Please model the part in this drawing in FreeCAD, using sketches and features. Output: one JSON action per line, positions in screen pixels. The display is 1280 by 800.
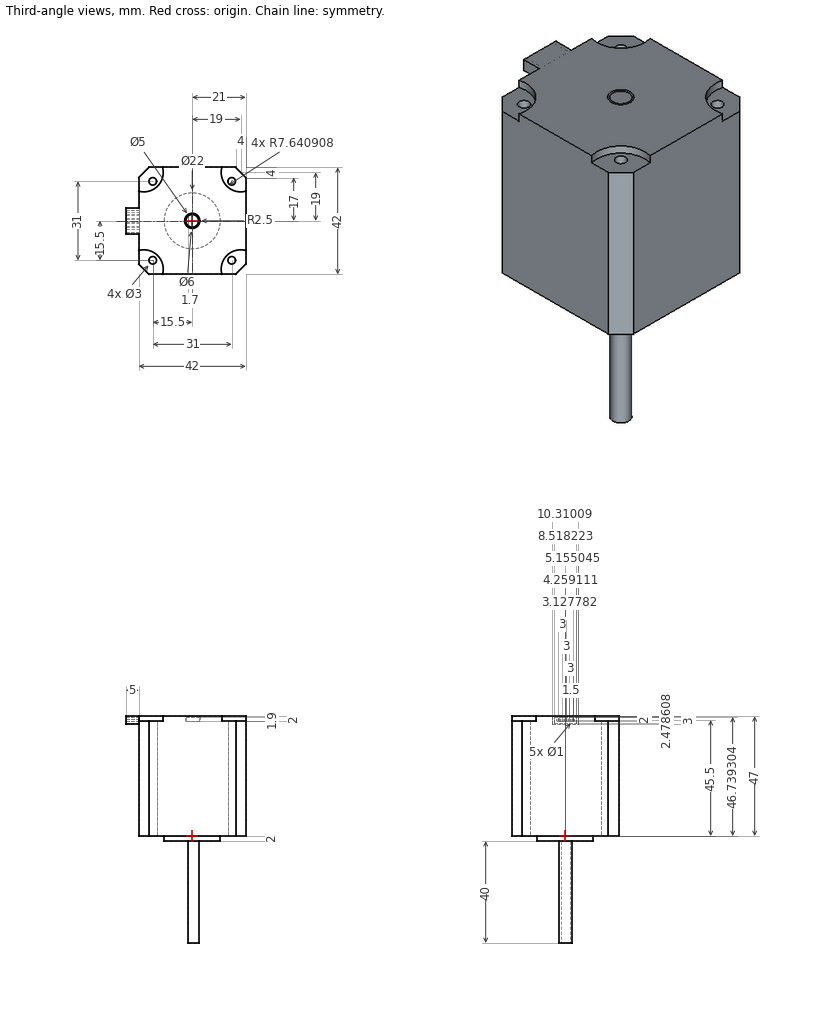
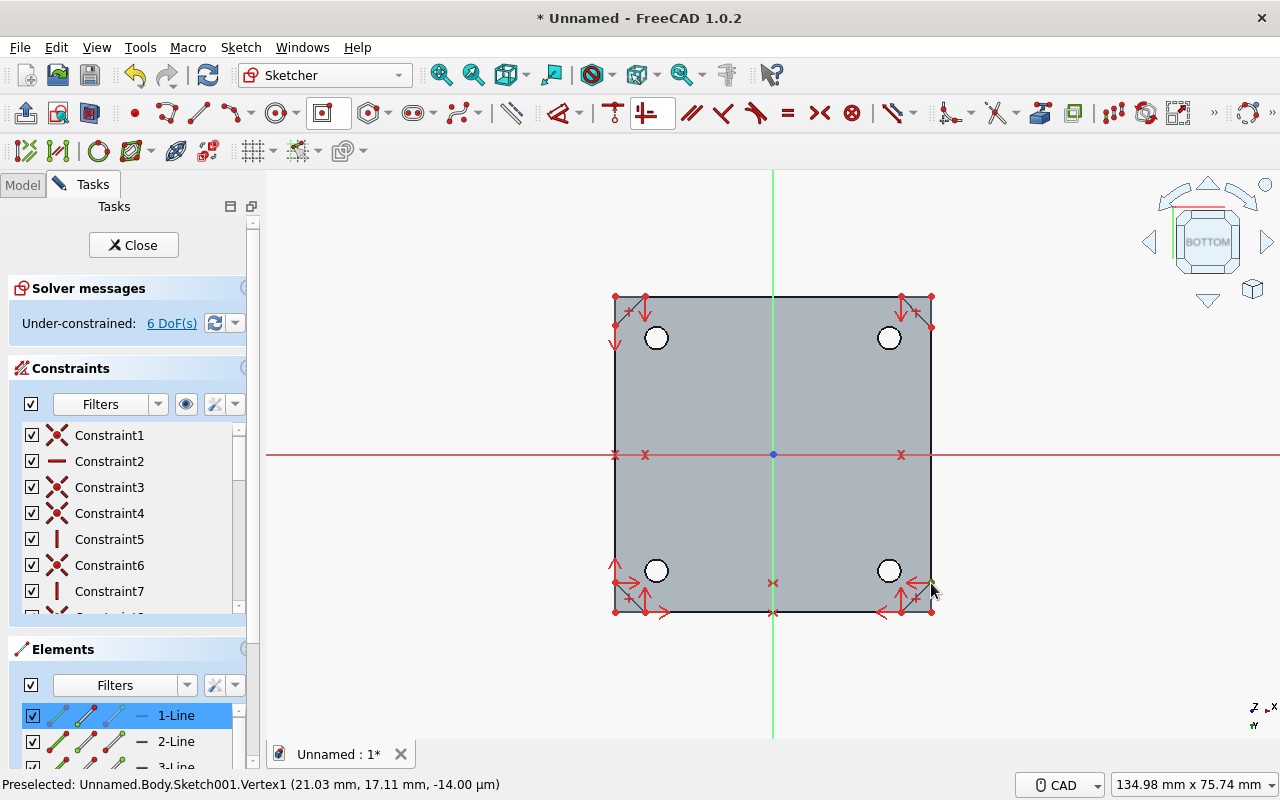
{"action": "left_click", "coordinate": [931, 328]}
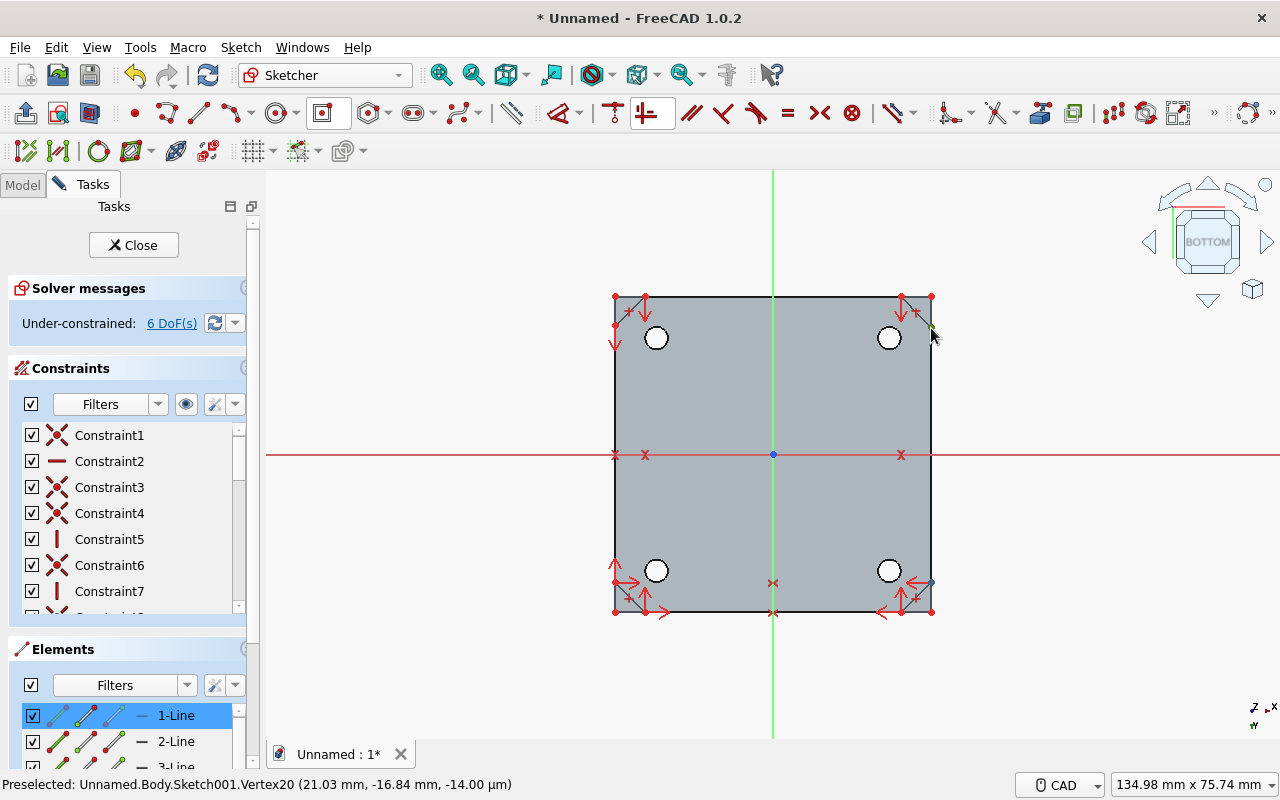
{"action": "left_click", "coordinate": [353, 454]}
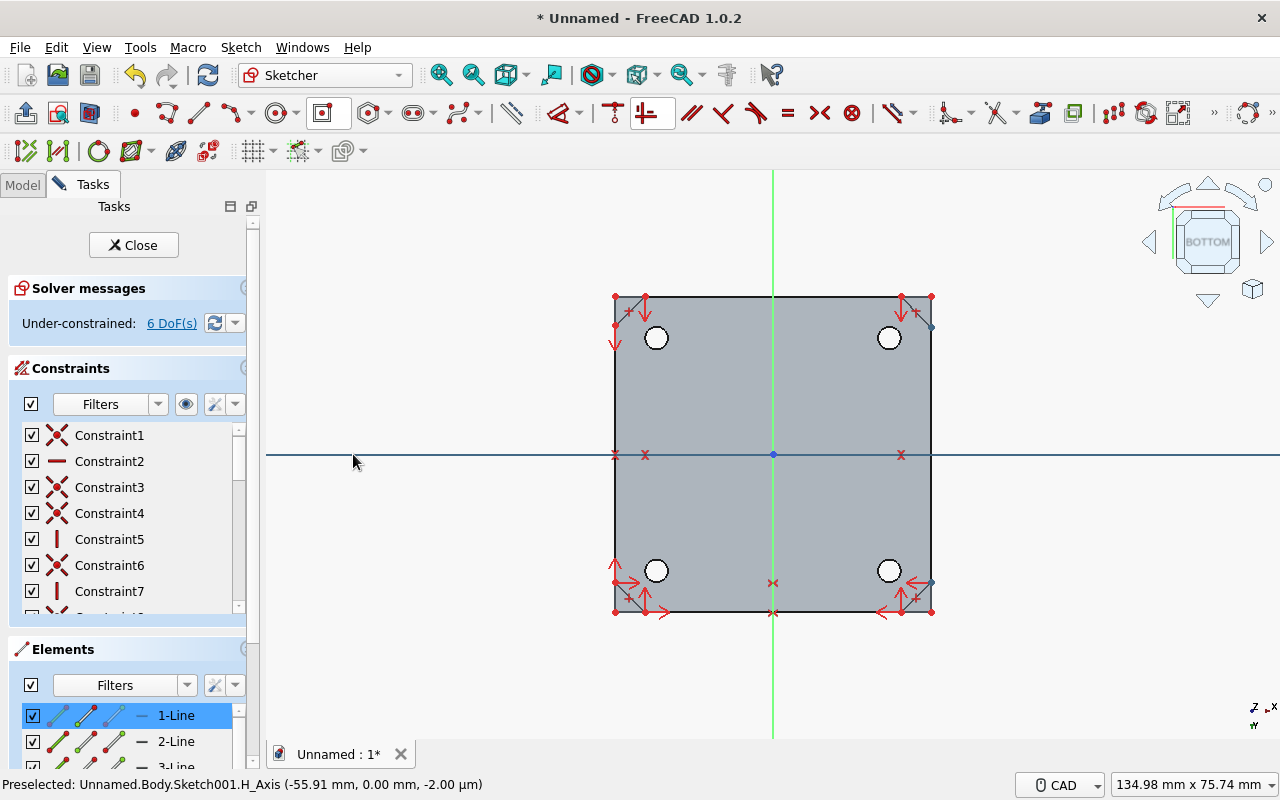
{"action": "left_click", "coordinate": [820, 114]}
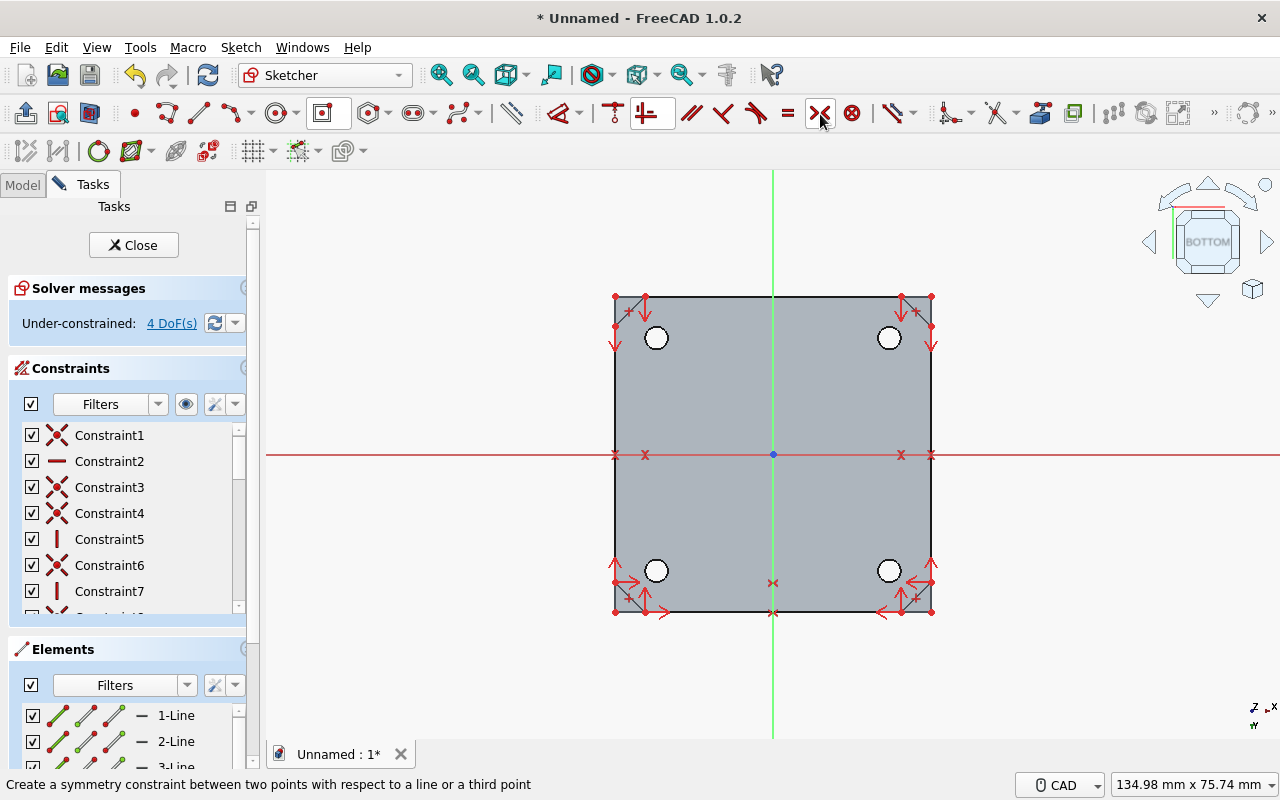
{"action": "left_click", "coordinate": [558, 114]}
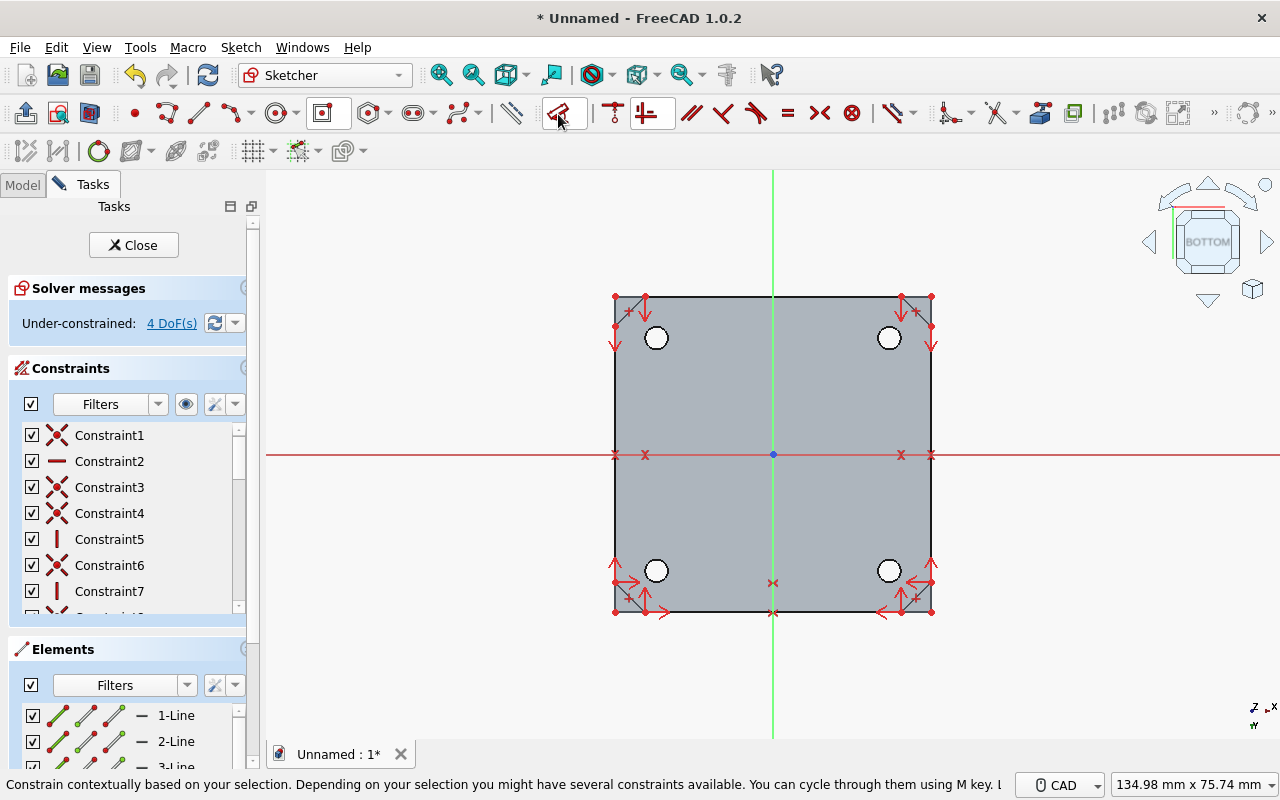
{"action": "scroll", "coordinate": [922, 612], "scroll_direction": "up", "scroll_amount": 3}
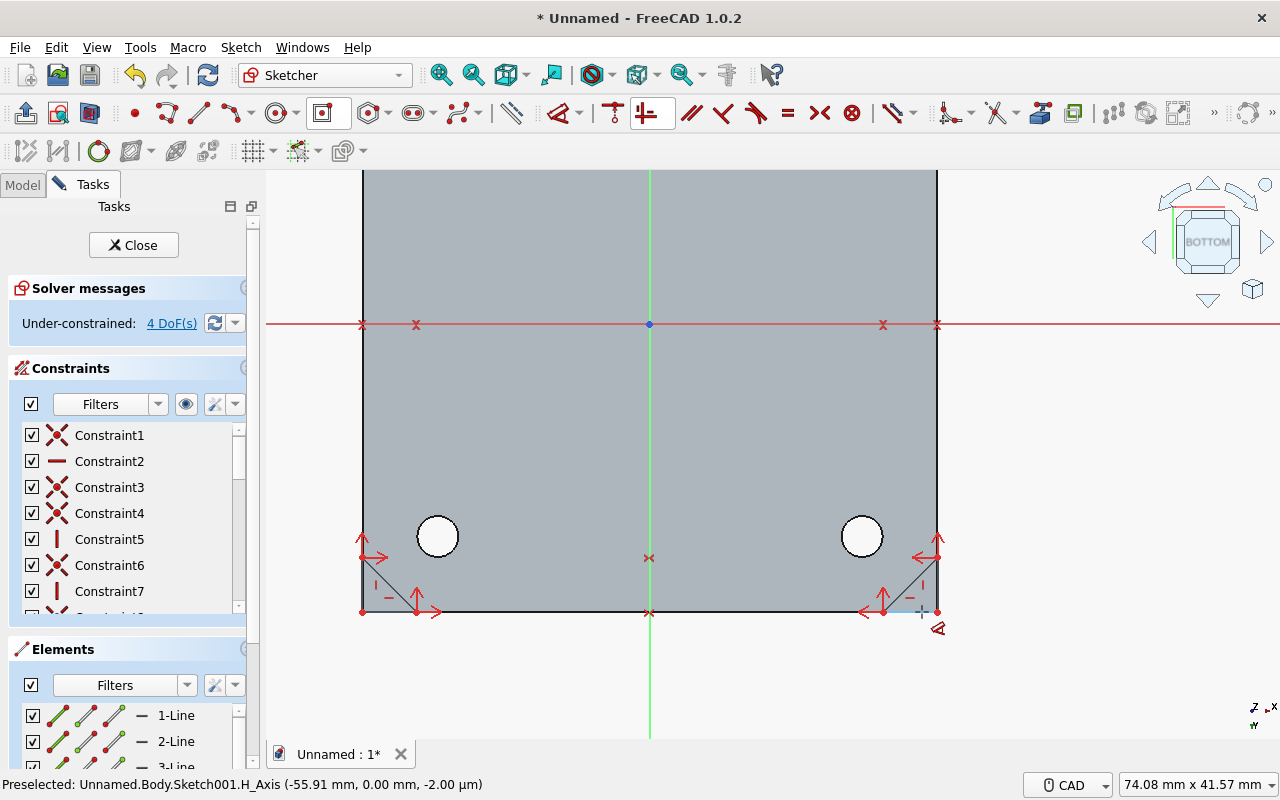
{"action": "left_click", "coordinate": [921, 612]}
{"action": "left_click", "coordinate": [911, 646]}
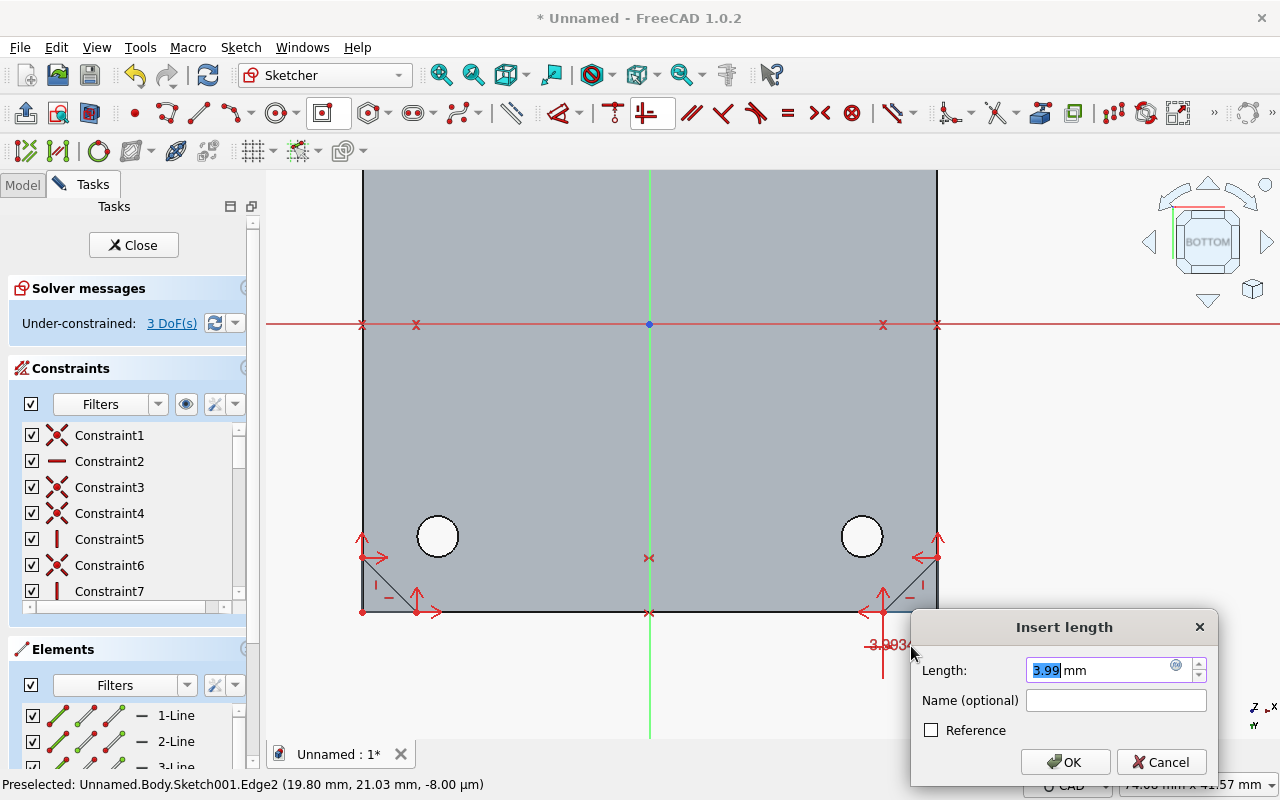
{"action": "type", "text": "4"}
{"action": "key", "text": "Return"}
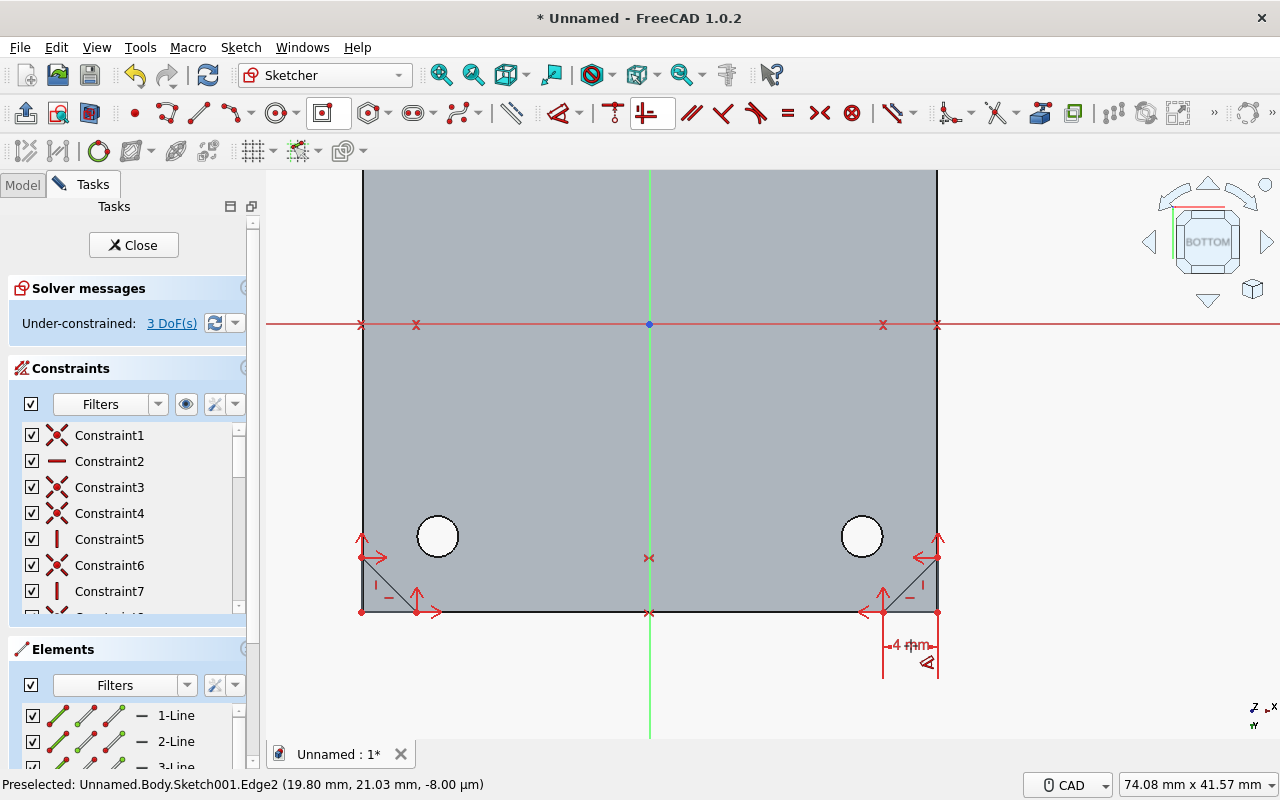
{"action": "left_click", "coordinate": [938, 596]}
{"action": "left_click", "coordinate": [972, 585]}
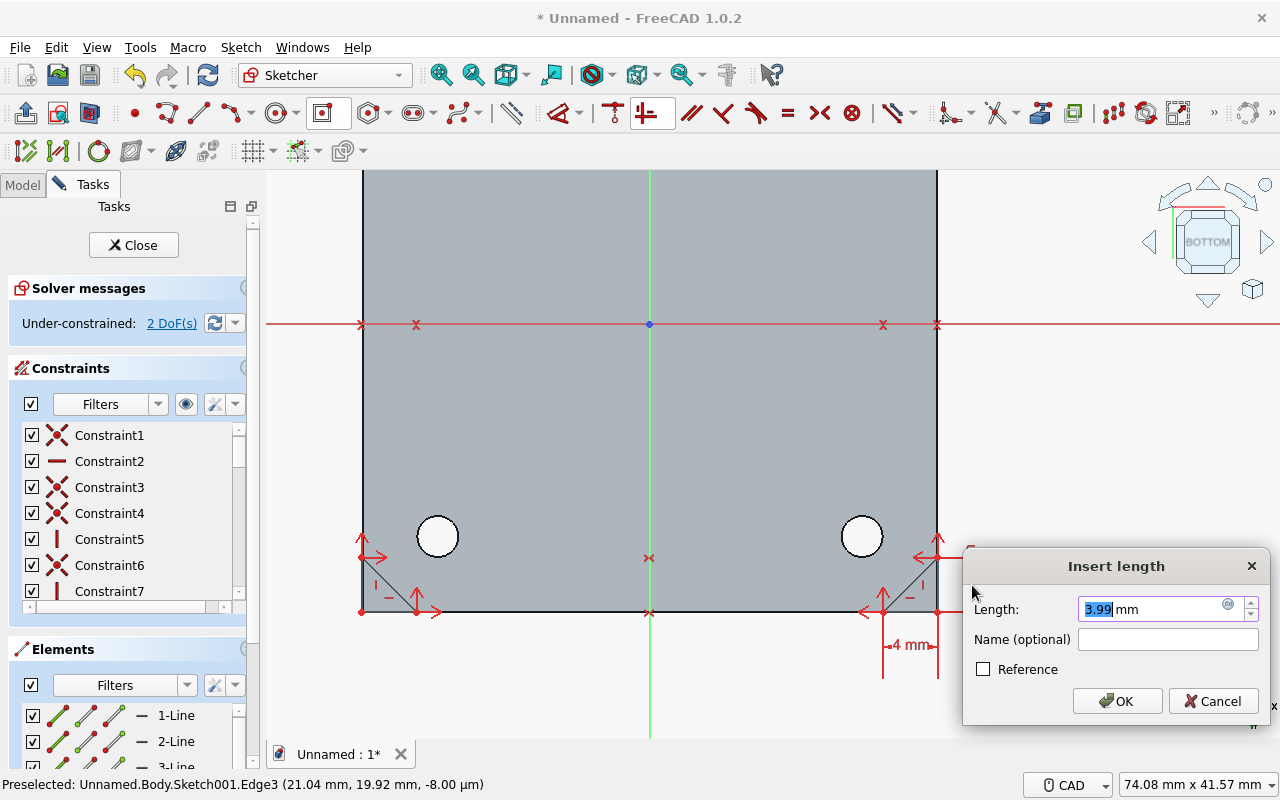
{"action": "type", "text": "4"}
{"action": "key", "text": "Return"}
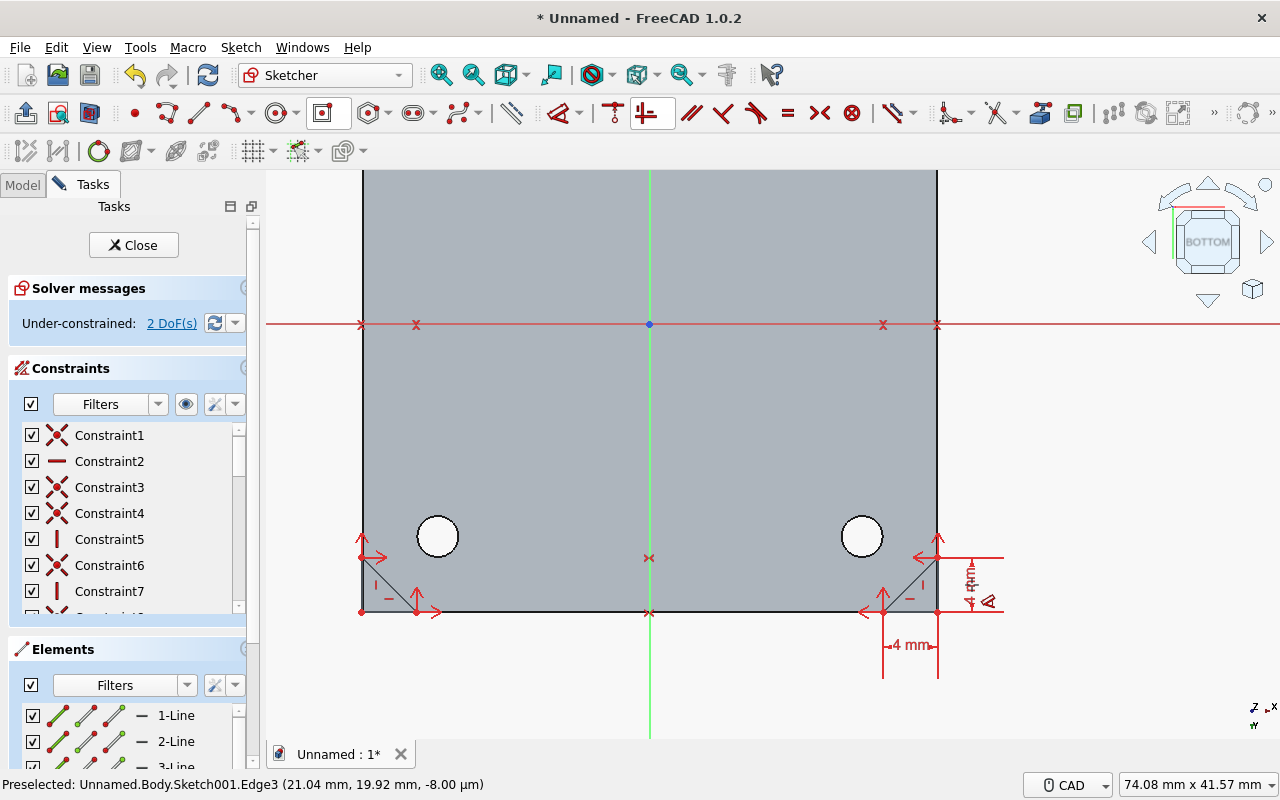
{"action": "left_click", "coordinate": [938, 558]}
{"action": "left_click", "coordinate": [794, 592]}